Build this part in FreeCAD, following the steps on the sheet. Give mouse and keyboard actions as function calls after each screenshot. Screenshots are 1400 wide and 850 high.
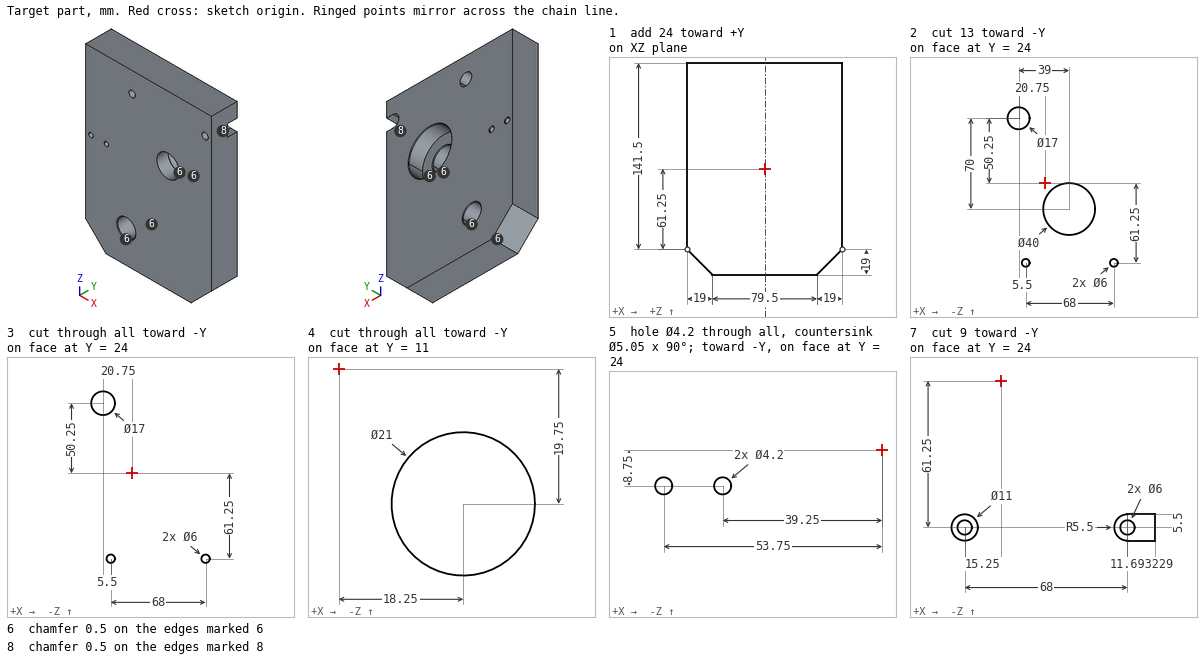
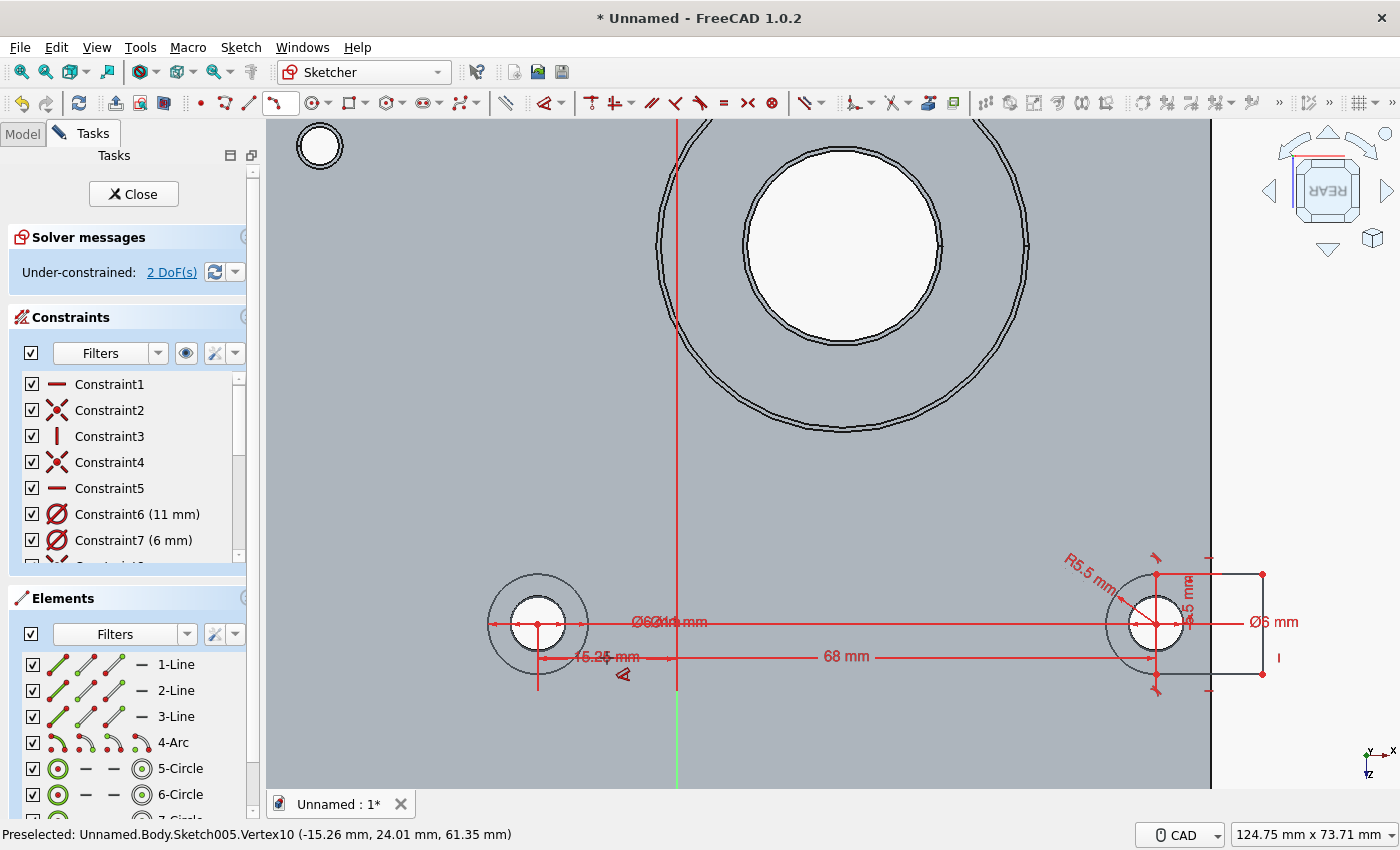
click(538, 624)
click(504, 386)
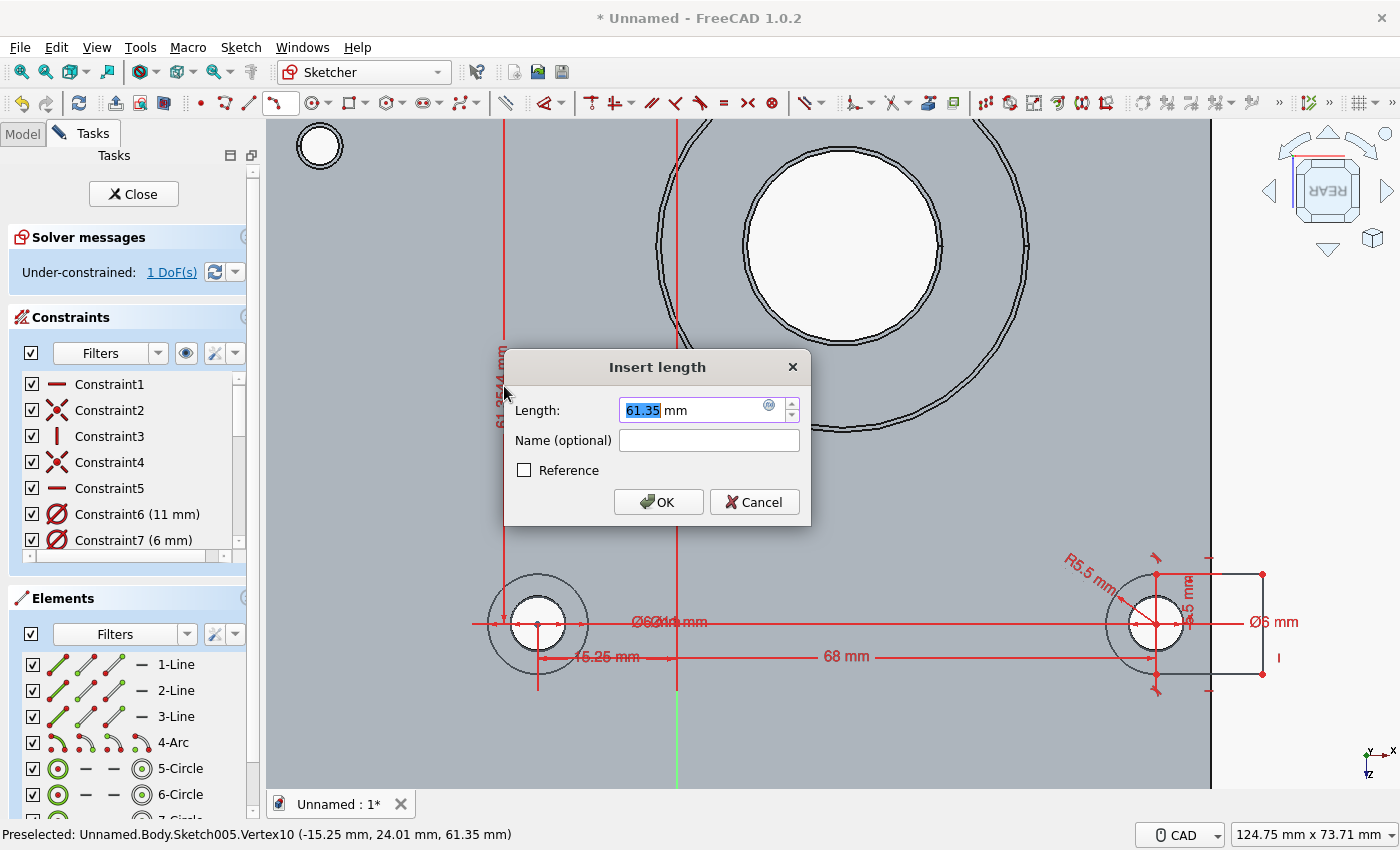
text(61.25)
key(Return)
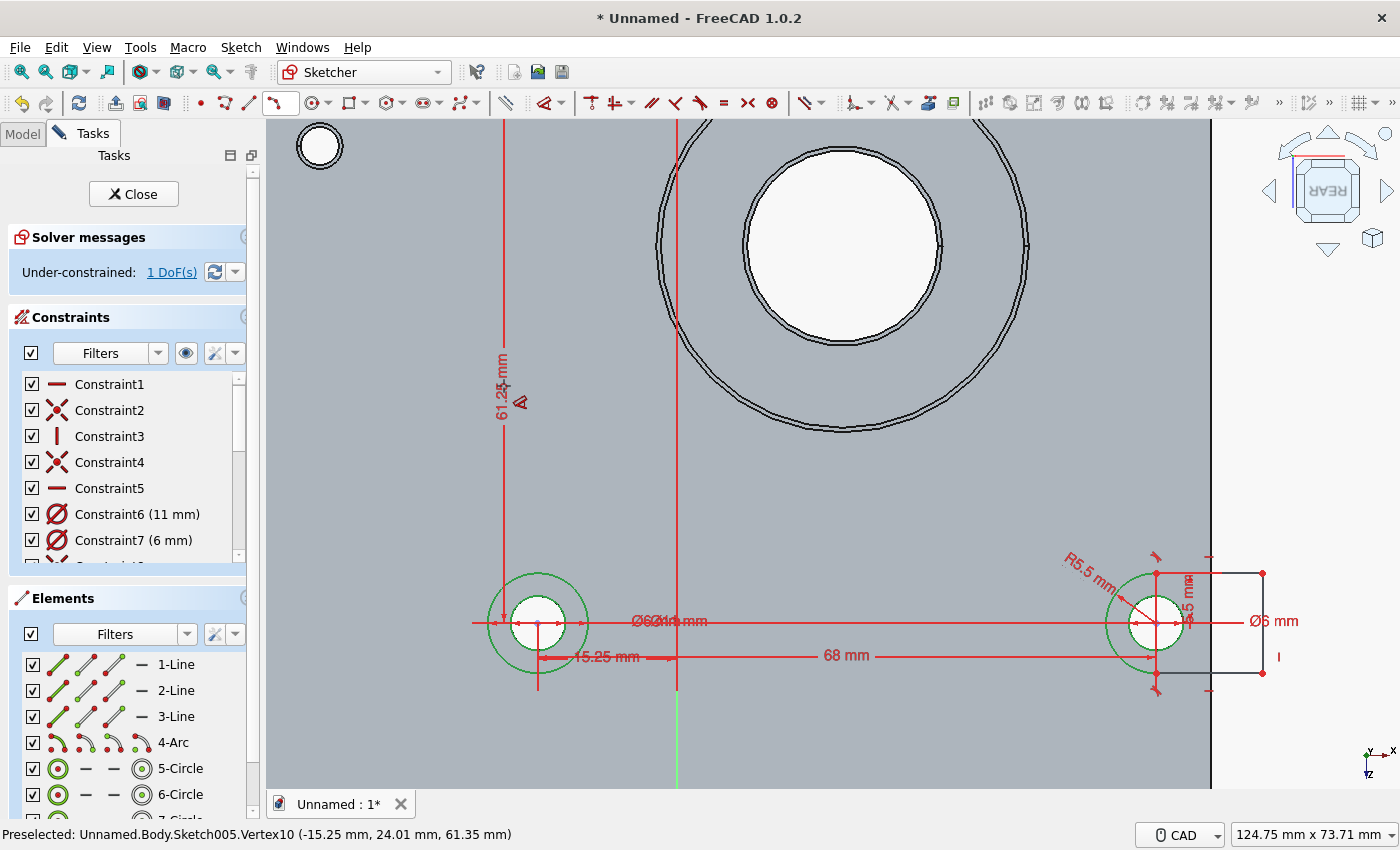
click(1188, 573)
click(1196, 539)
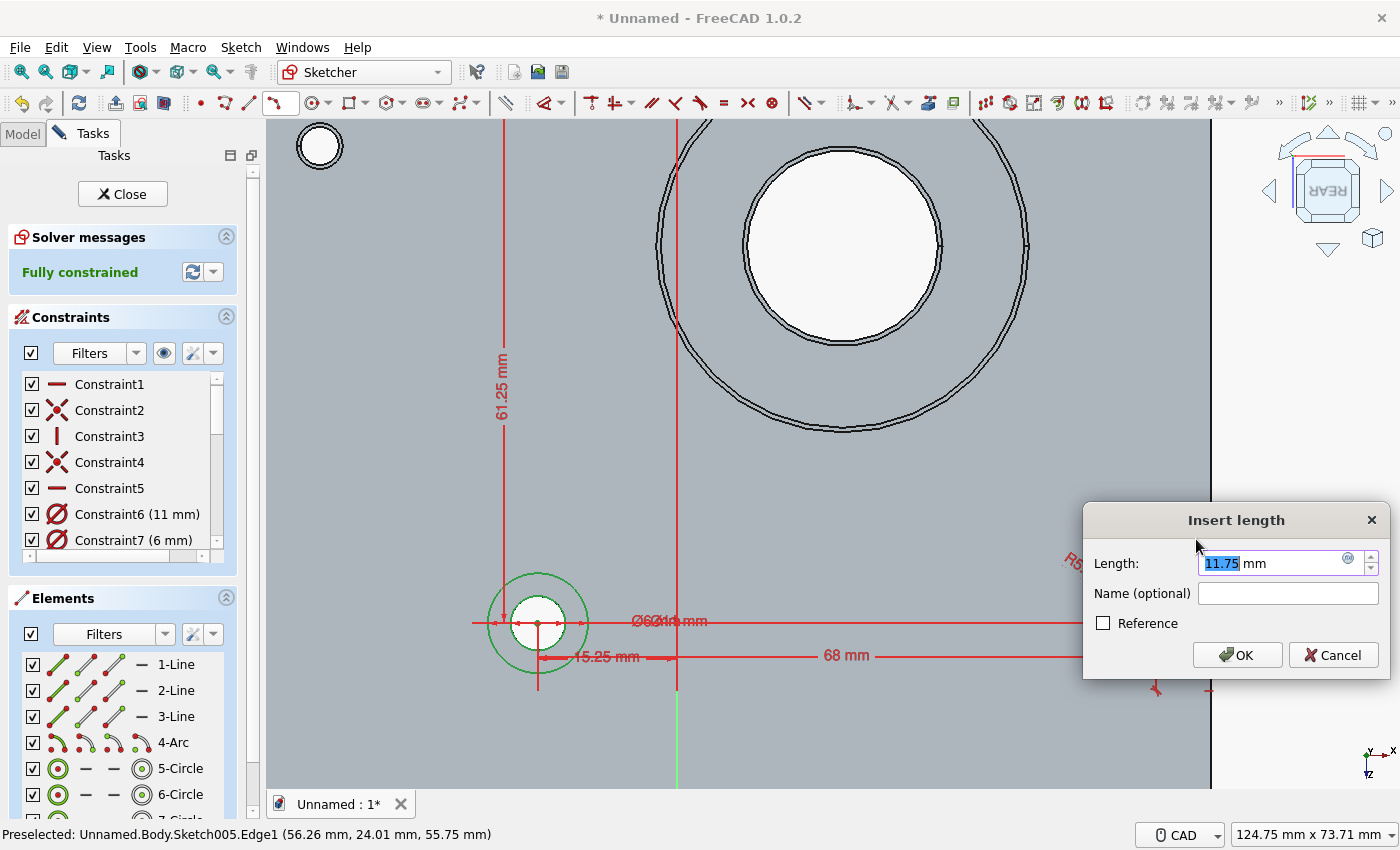
text(11.693229)
key(Return)
key(Escape)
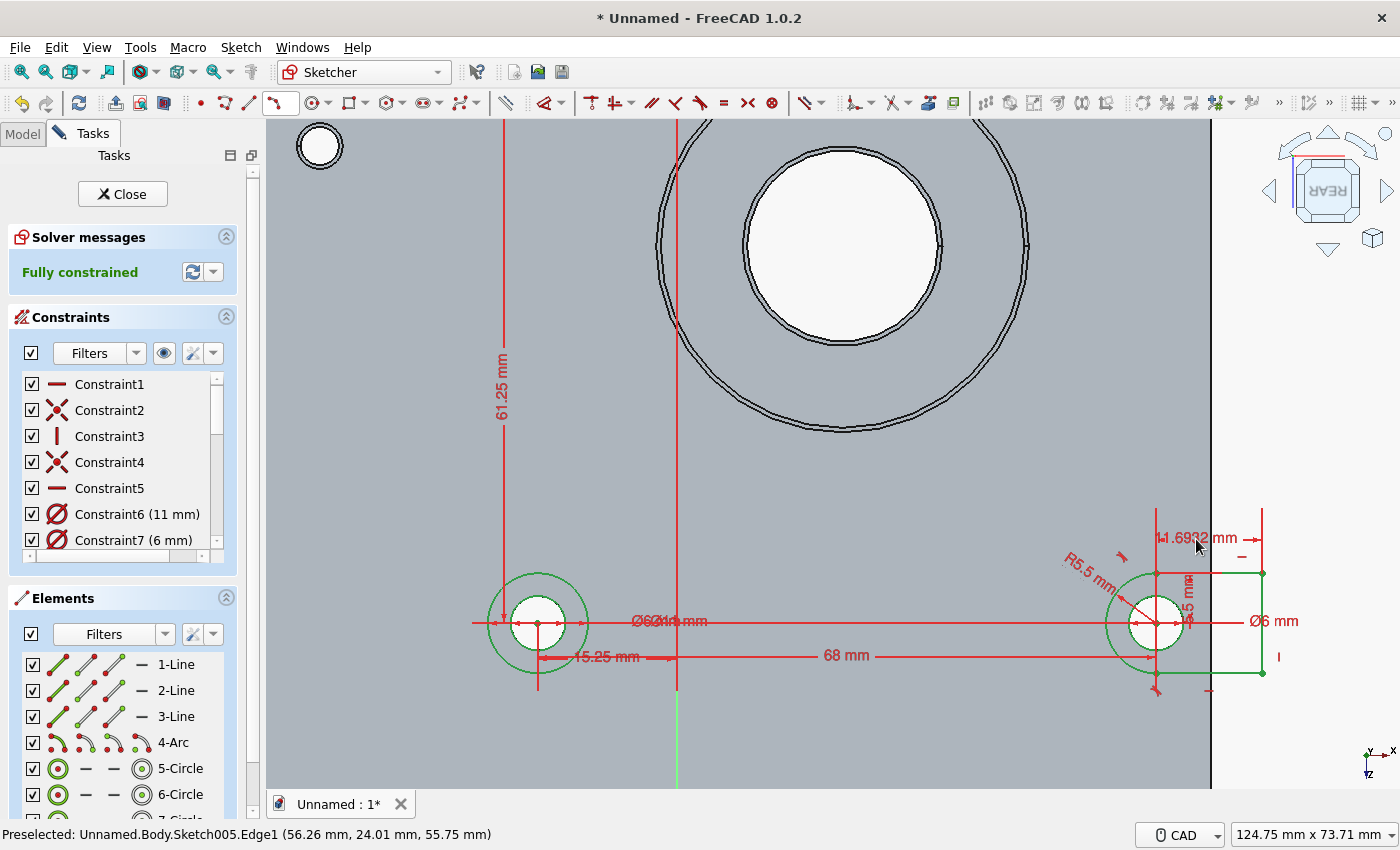
click(123, 194)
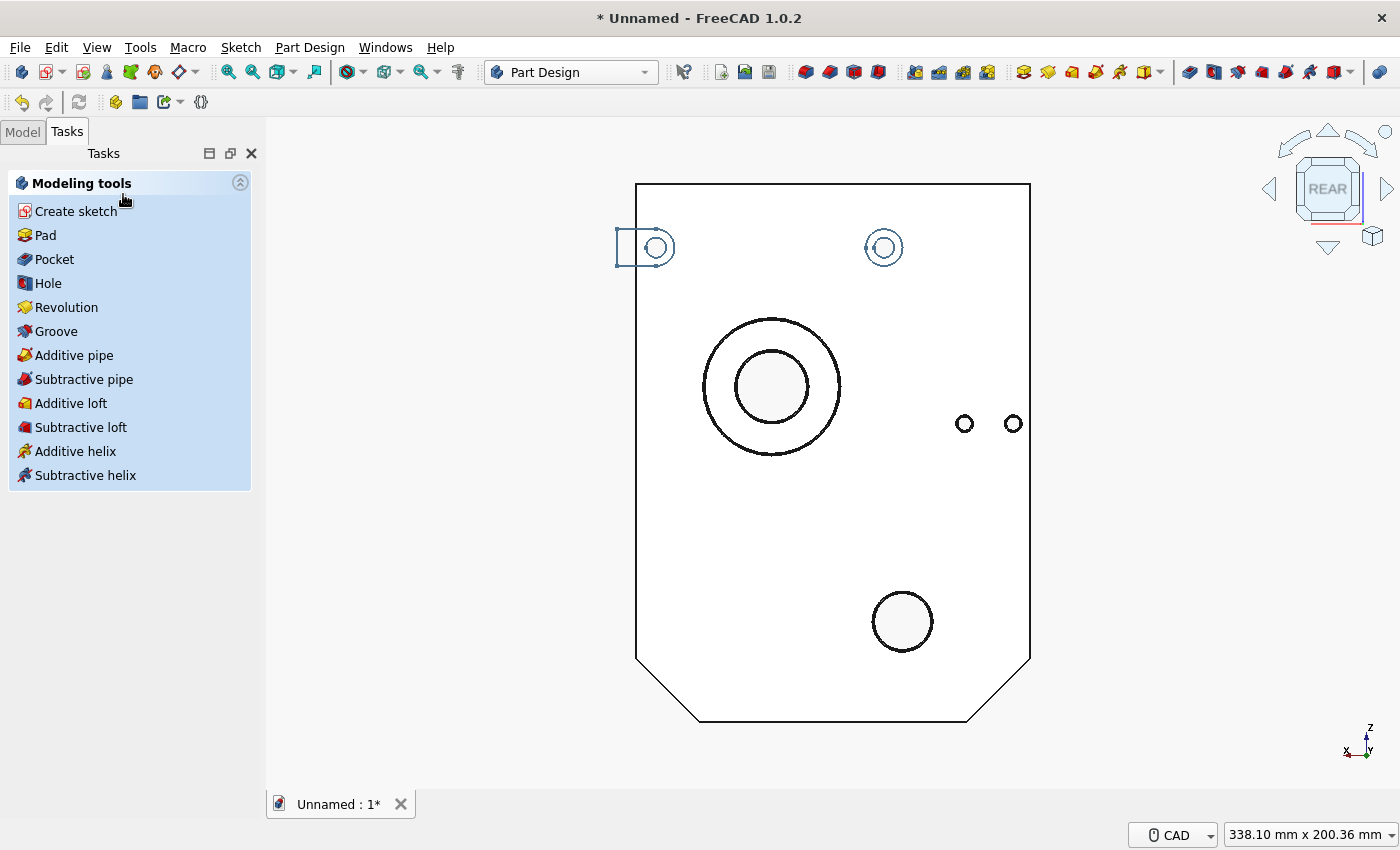
click(1190, 72)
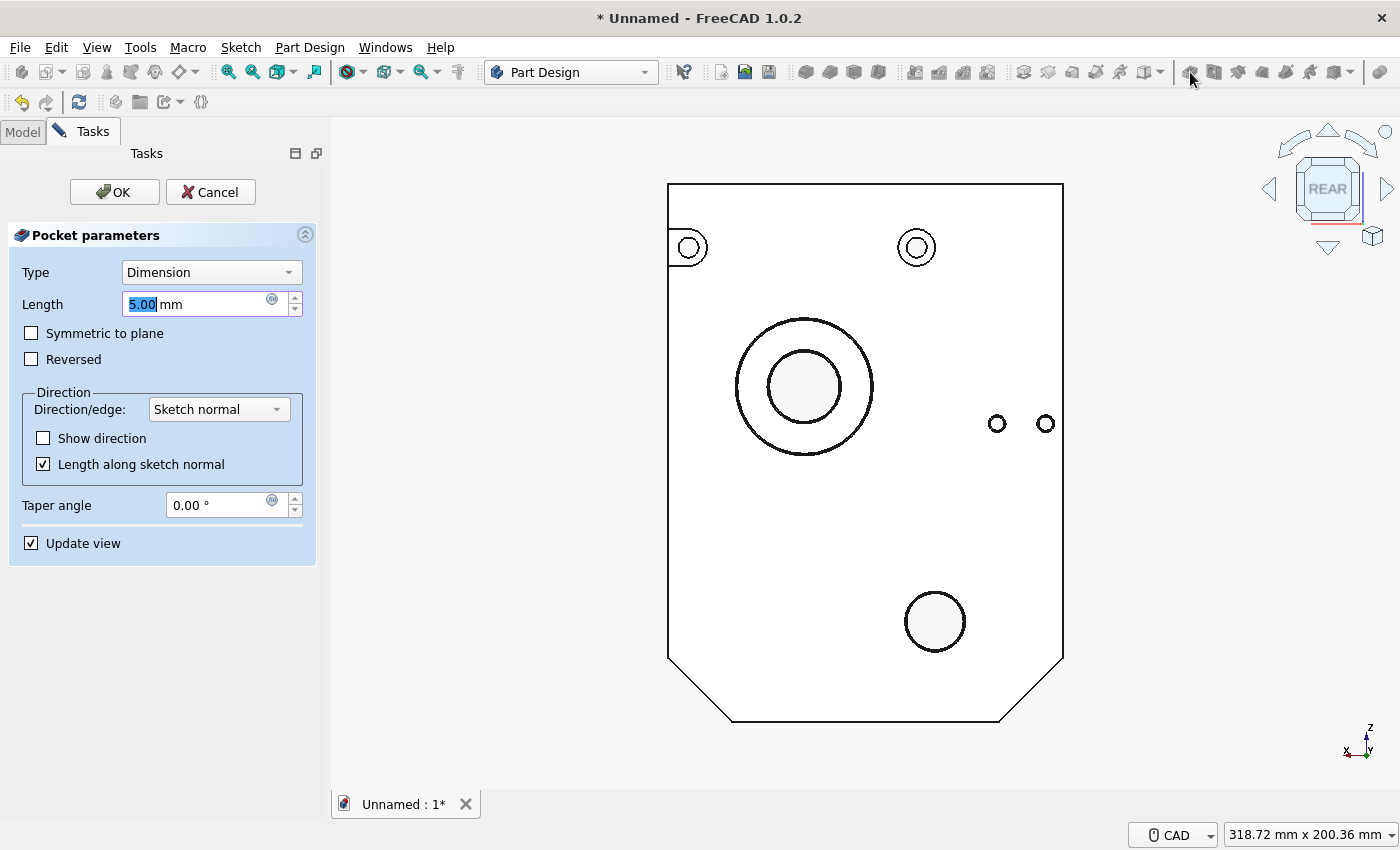
text(9)
key(Tab)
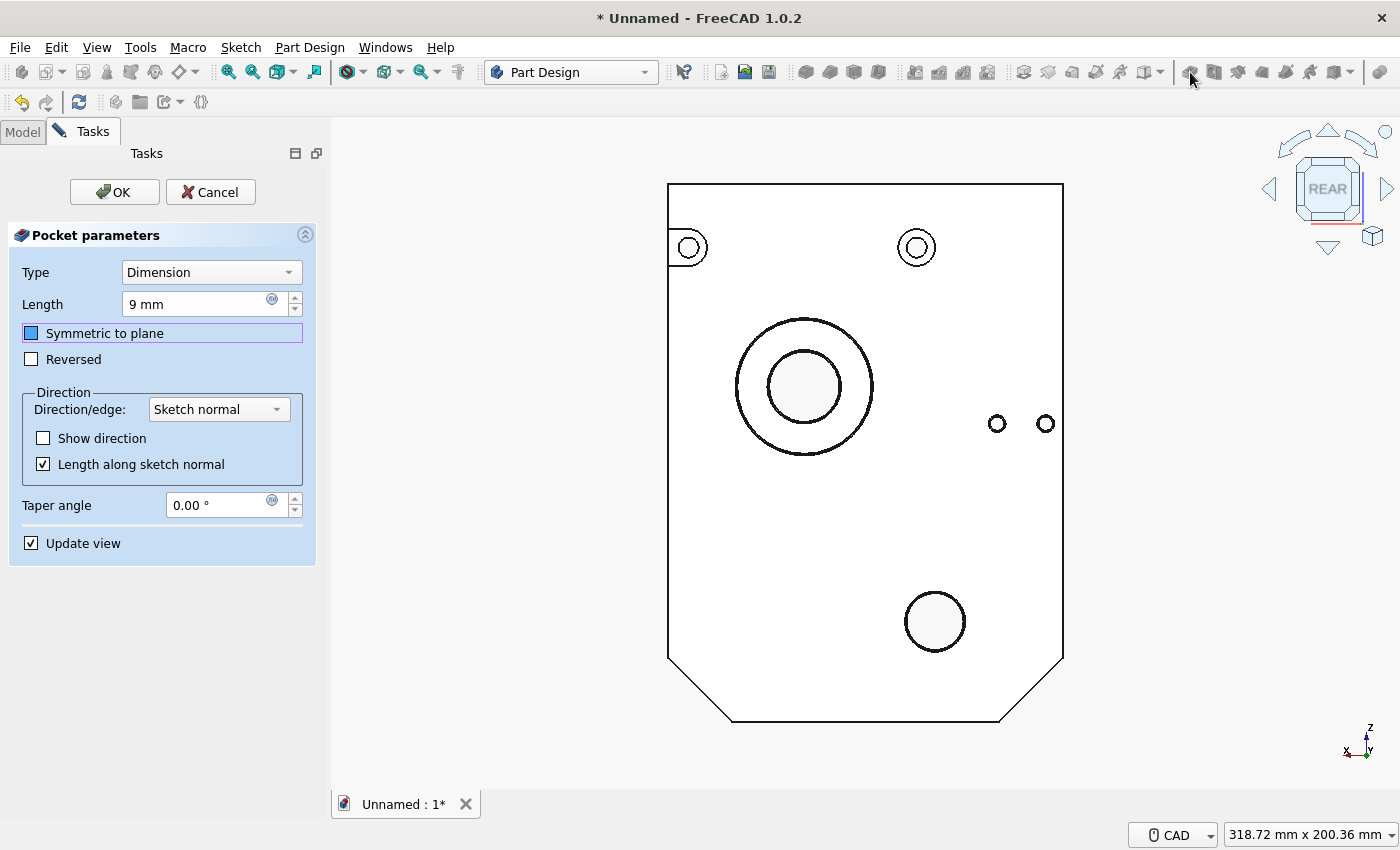
click(115, 192)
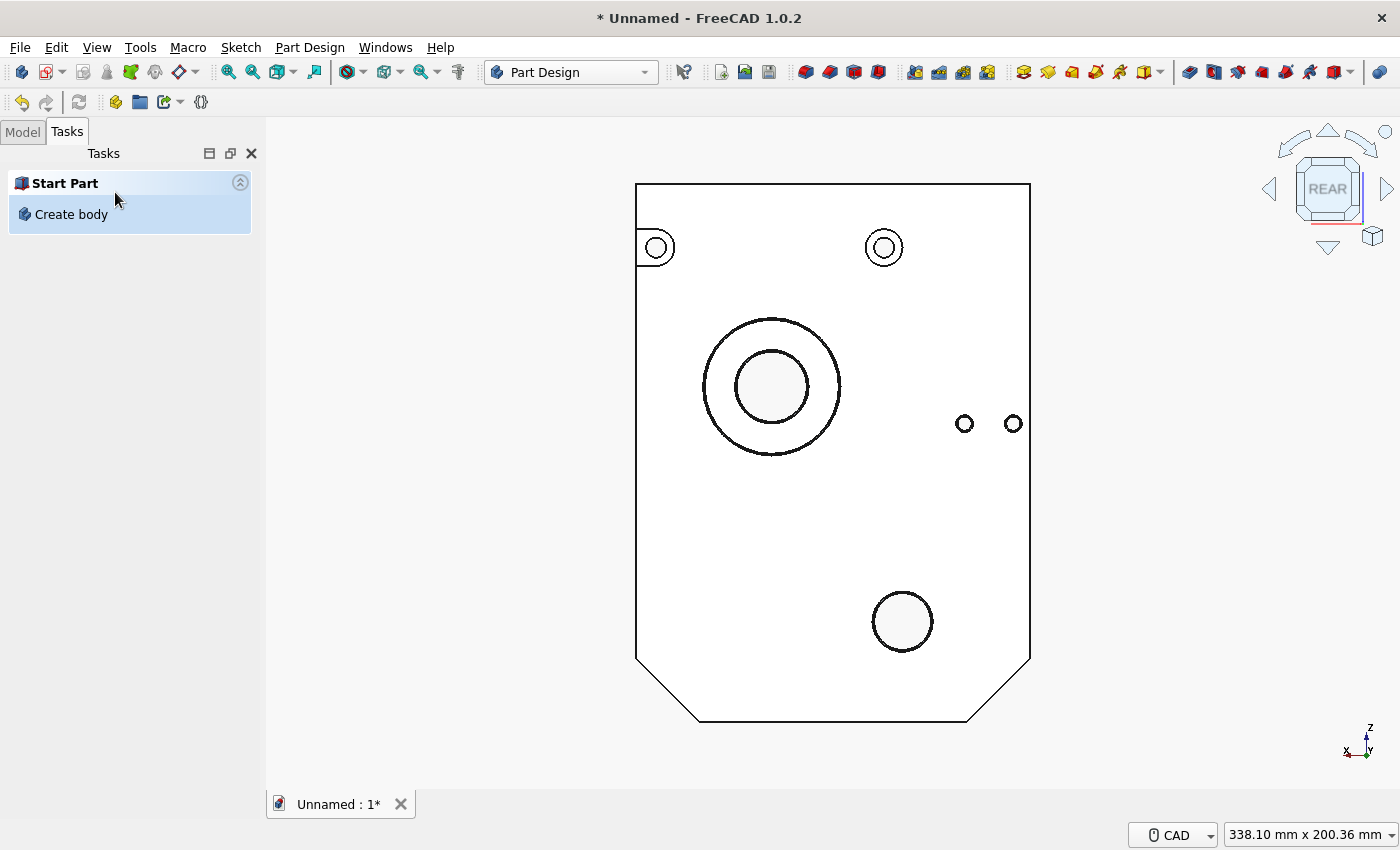
click(666, 247)